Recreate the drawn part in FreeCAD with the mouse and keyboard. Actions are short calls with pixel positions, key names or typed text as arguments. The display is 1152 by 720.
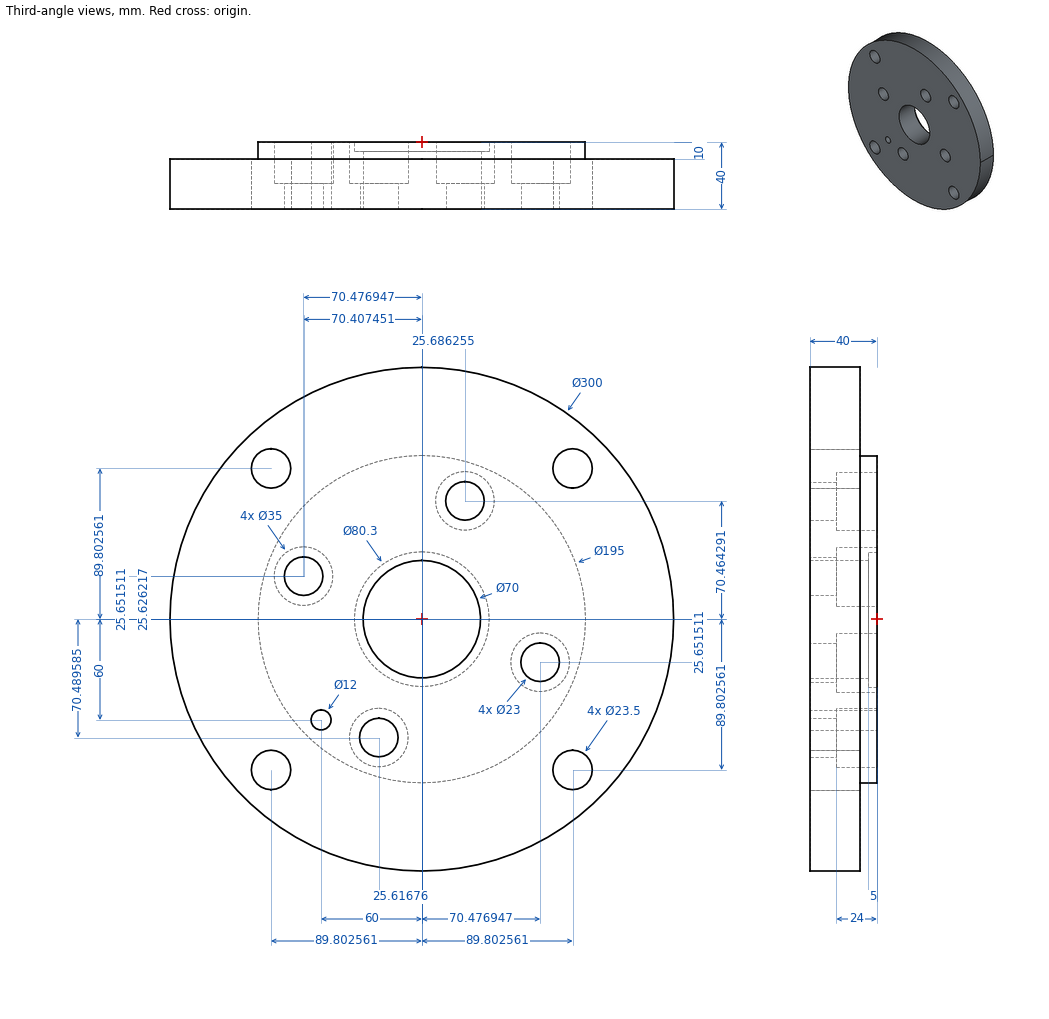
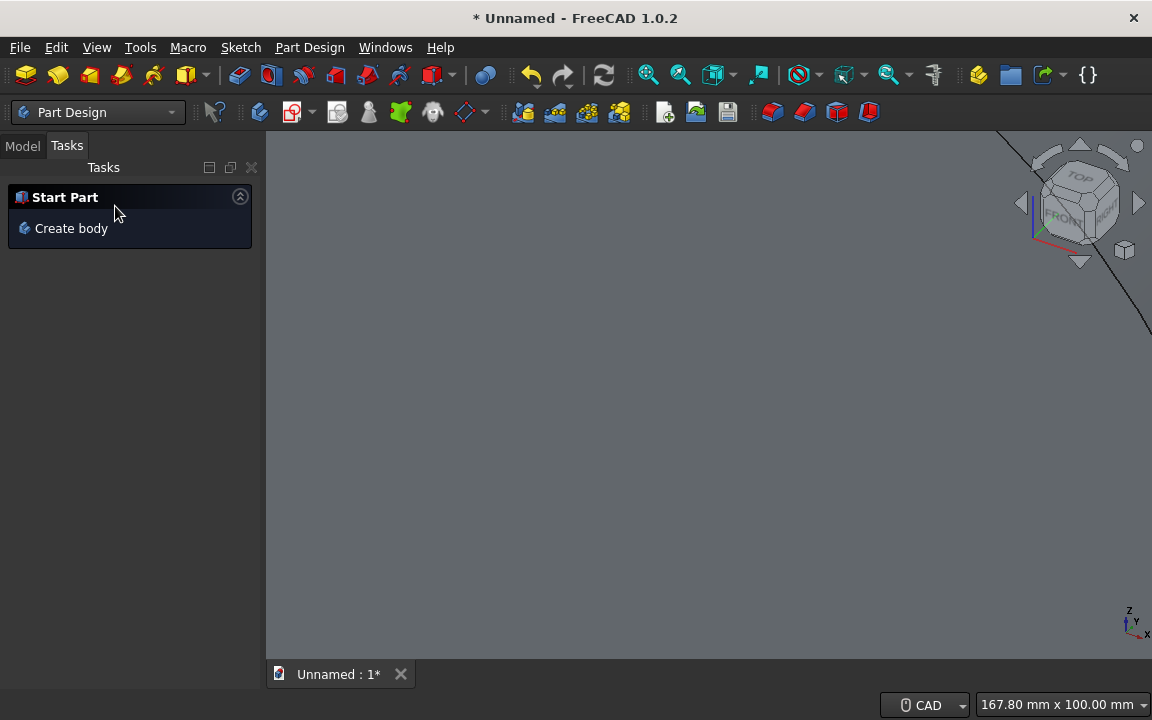
click(650, 76)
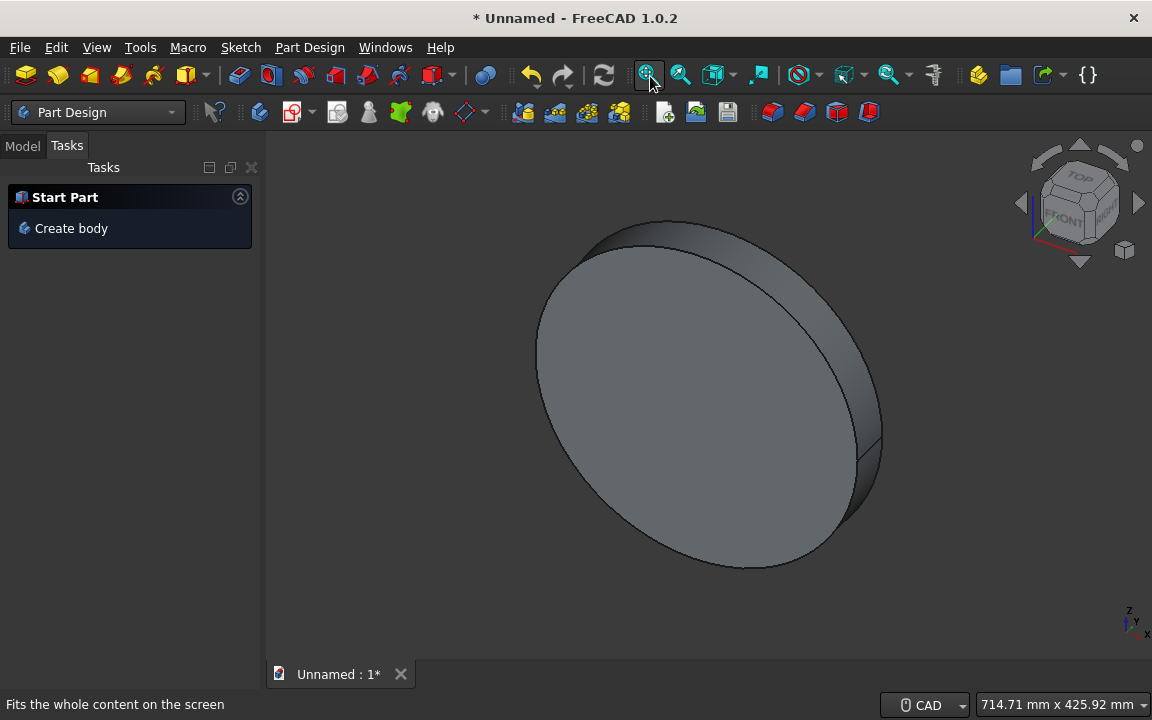
key(4)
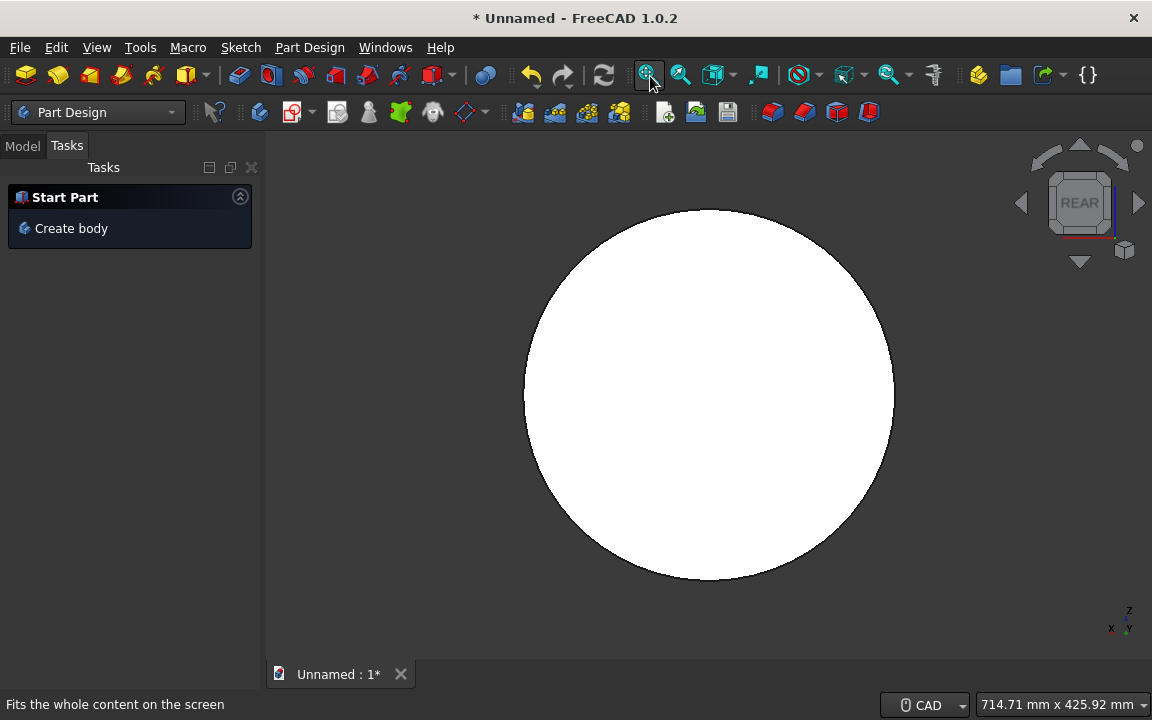
click(709, 394)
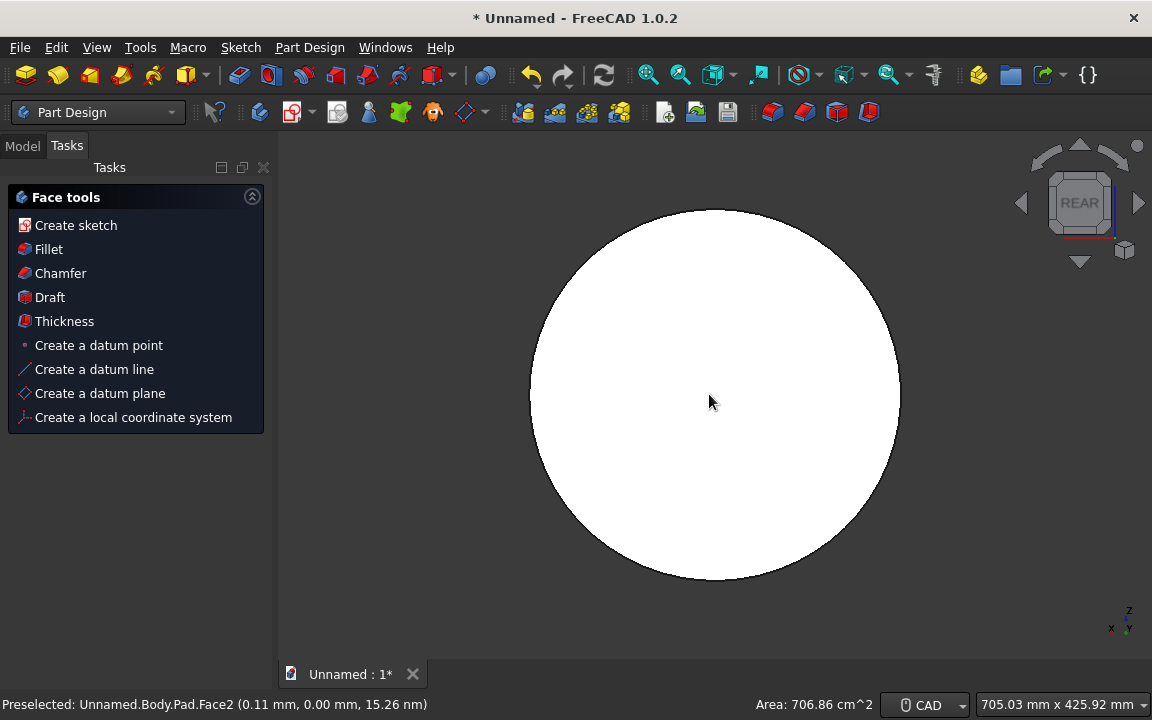
click(292, 112)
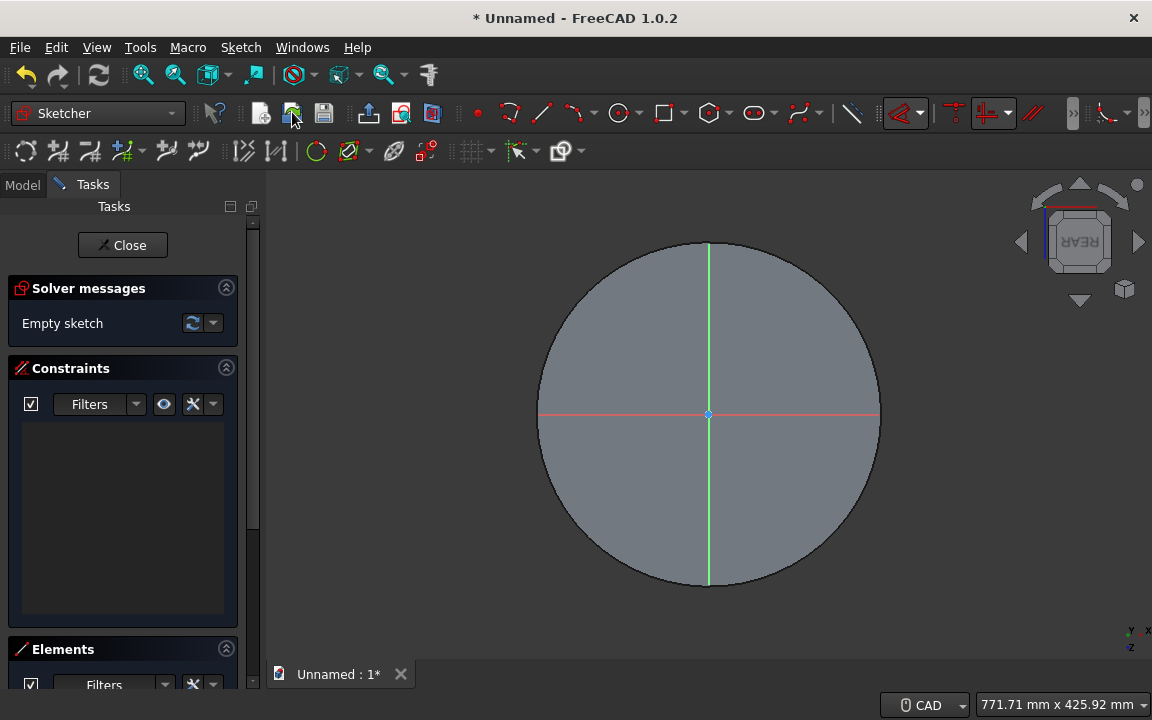
scroll(731, 414, up, 7)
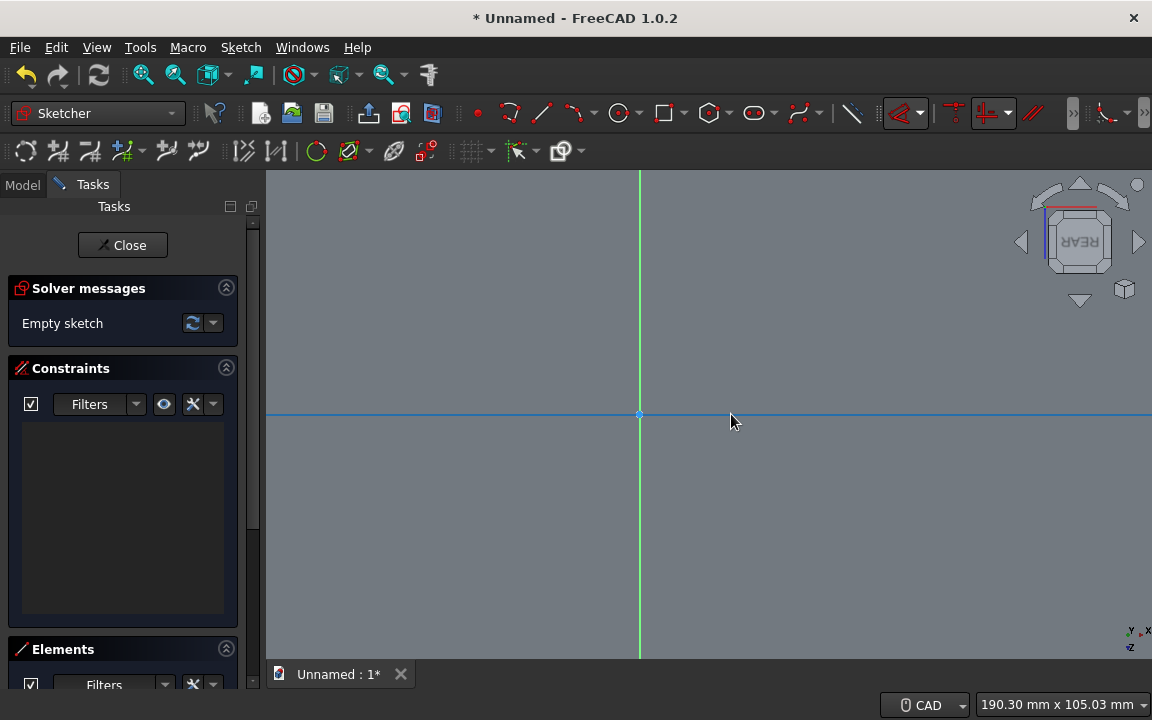
click(620, 114)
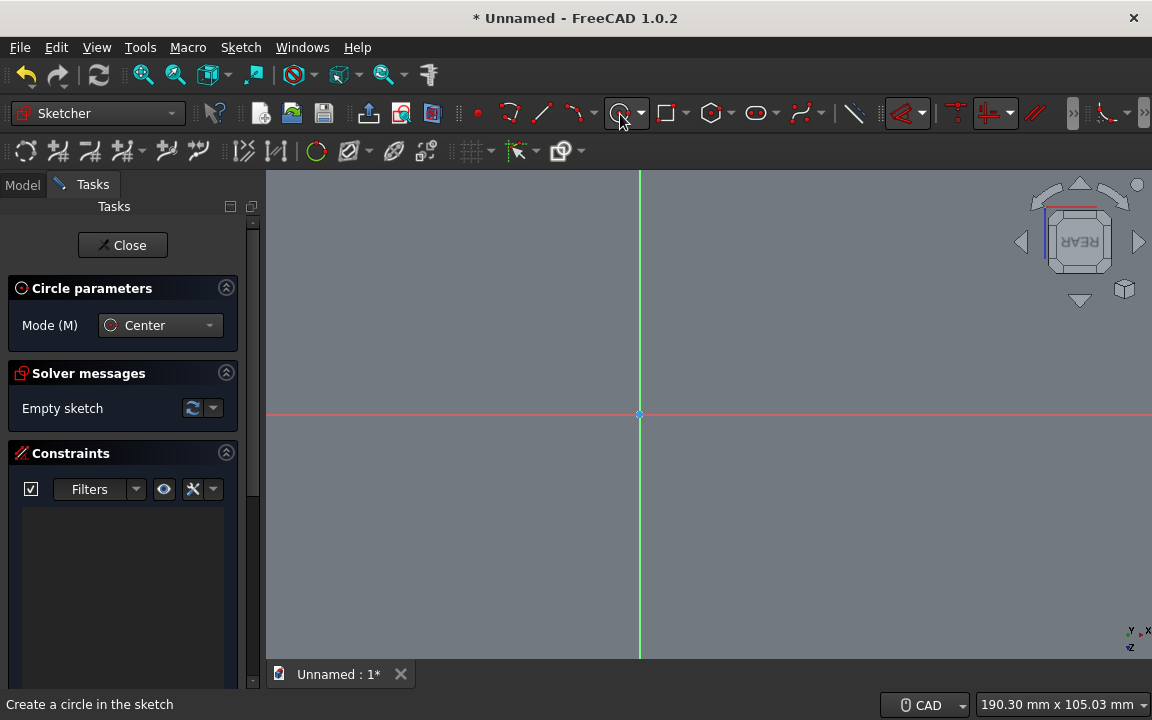
click(640, 414)
move(755, 299)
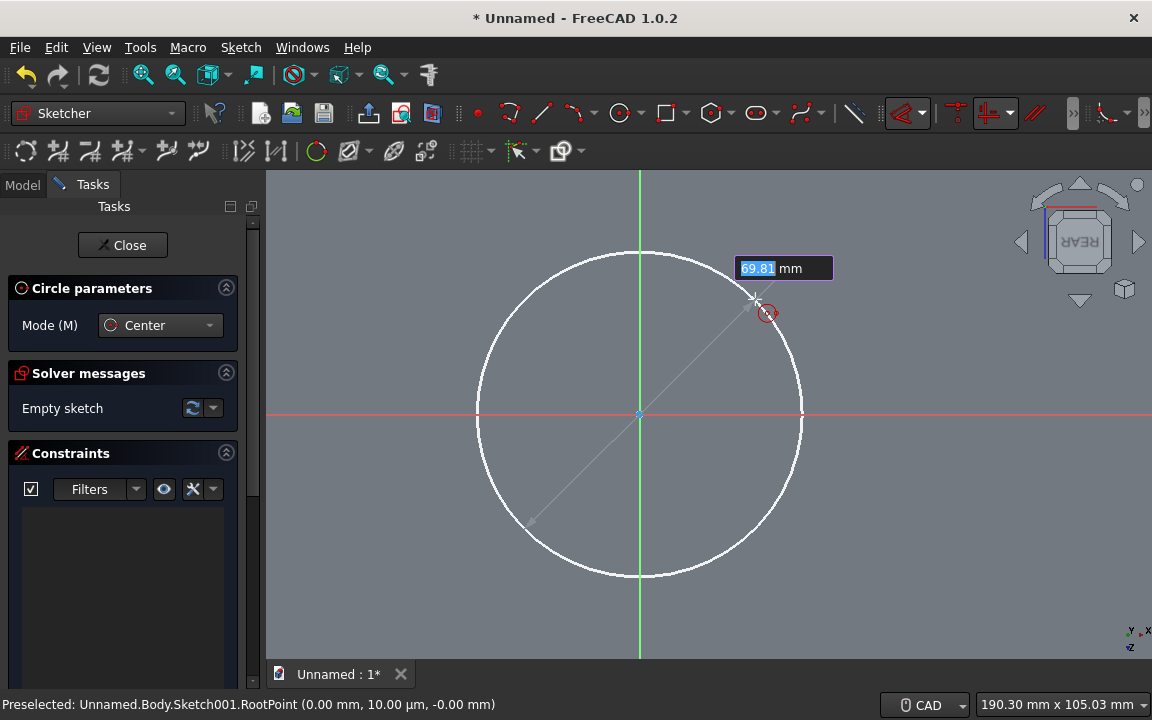
text(70)
key(Return)
key(Escape)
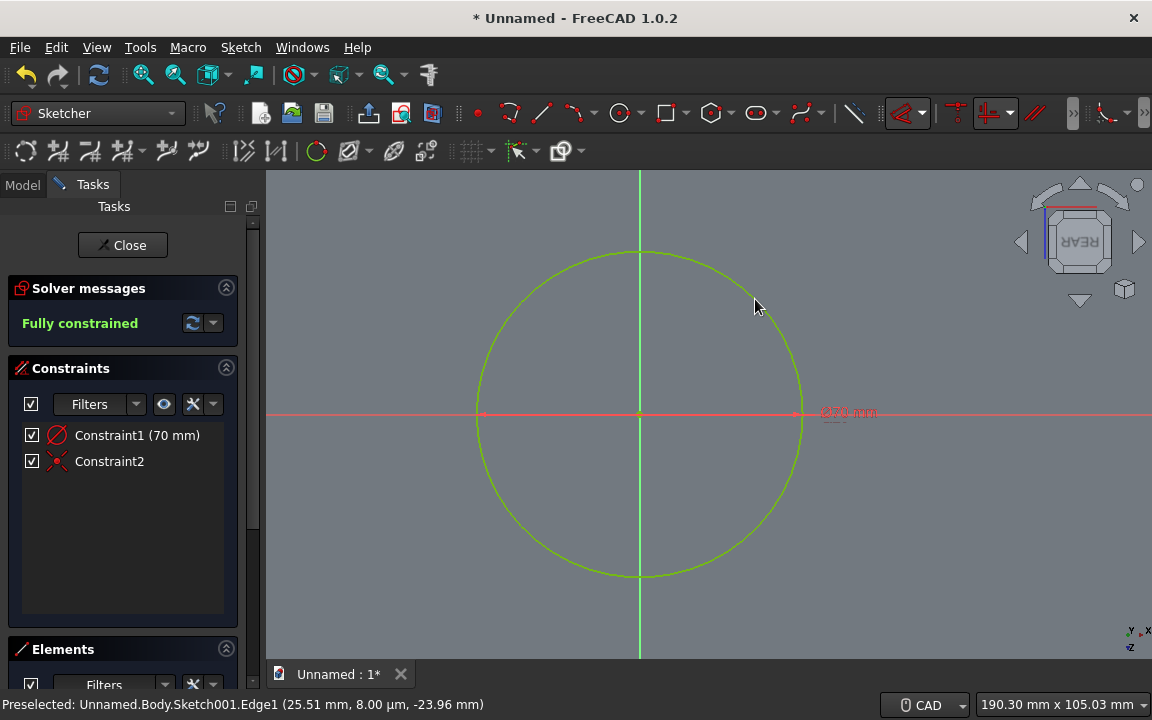
click(123, 245)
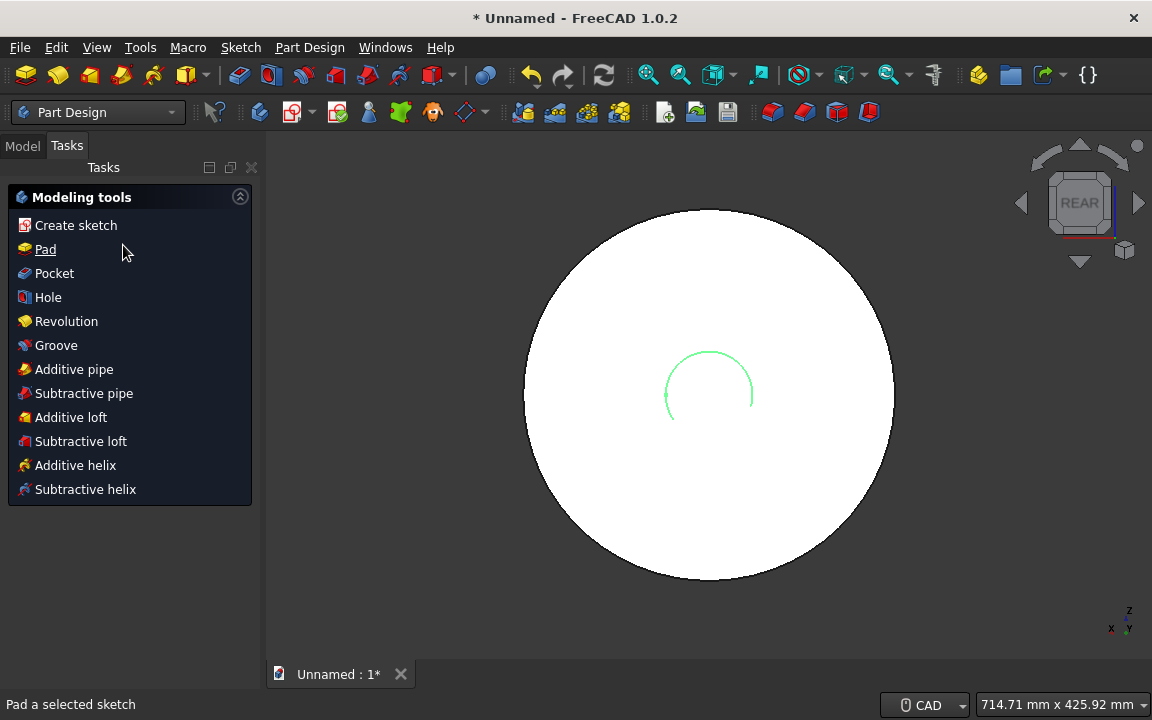
click(240, 76)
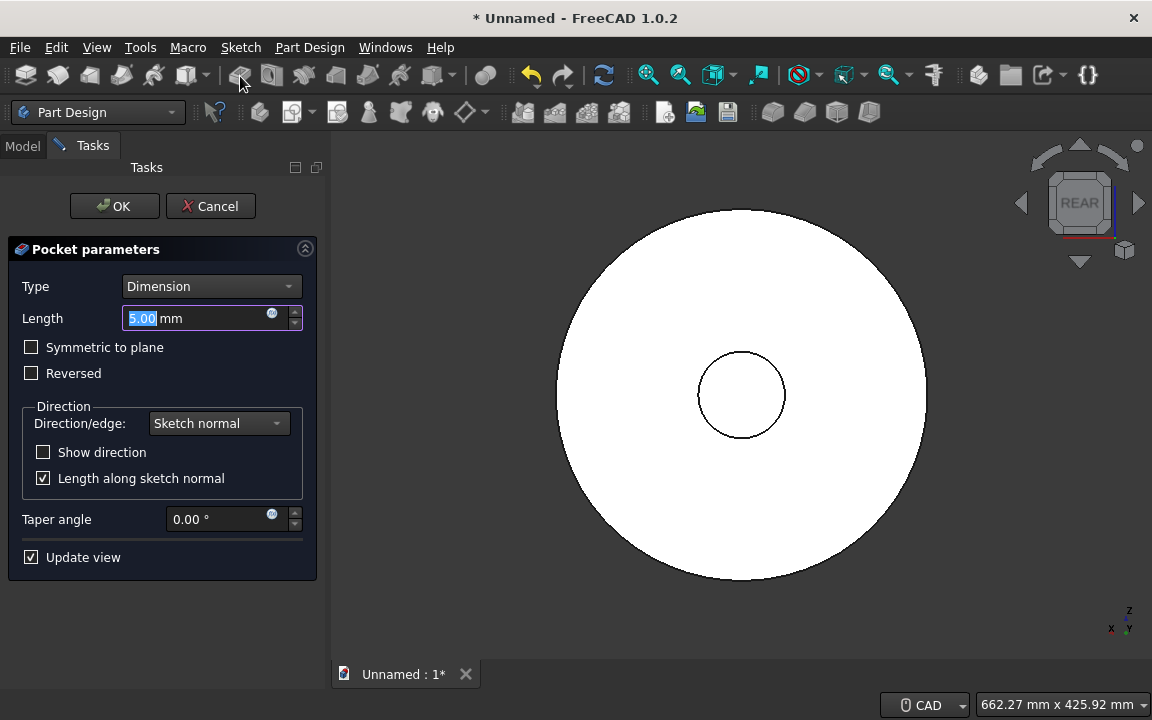
text(40)
key(Tab)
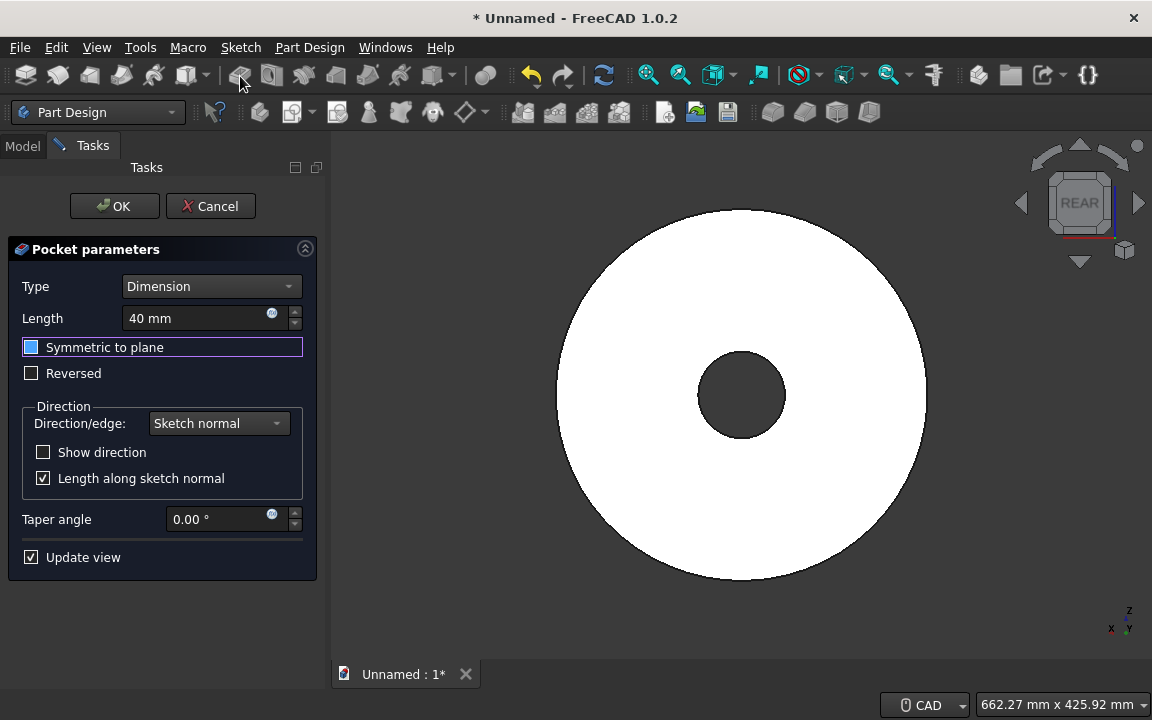
click(115, 206)